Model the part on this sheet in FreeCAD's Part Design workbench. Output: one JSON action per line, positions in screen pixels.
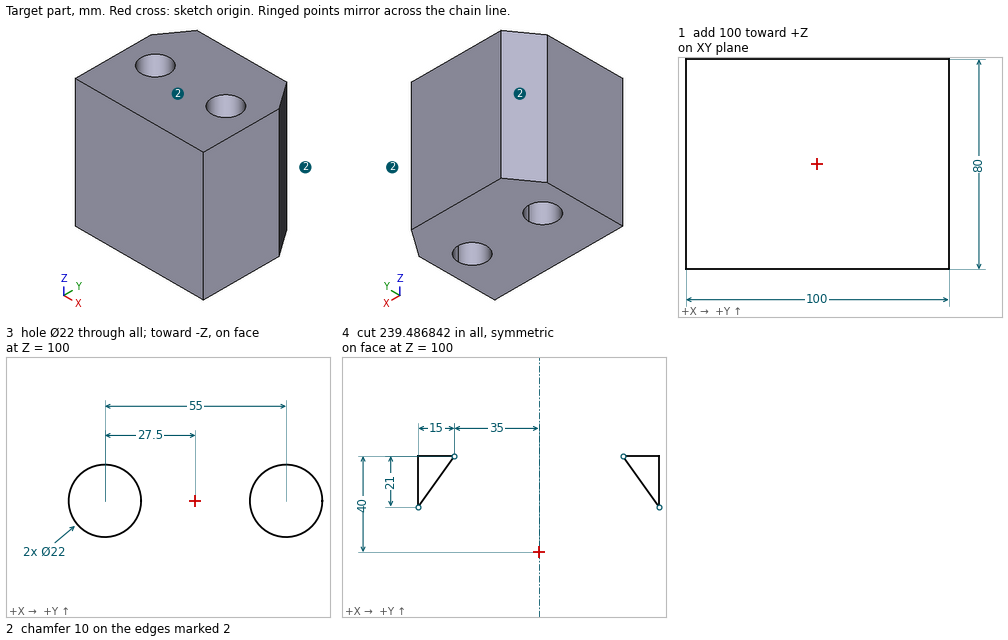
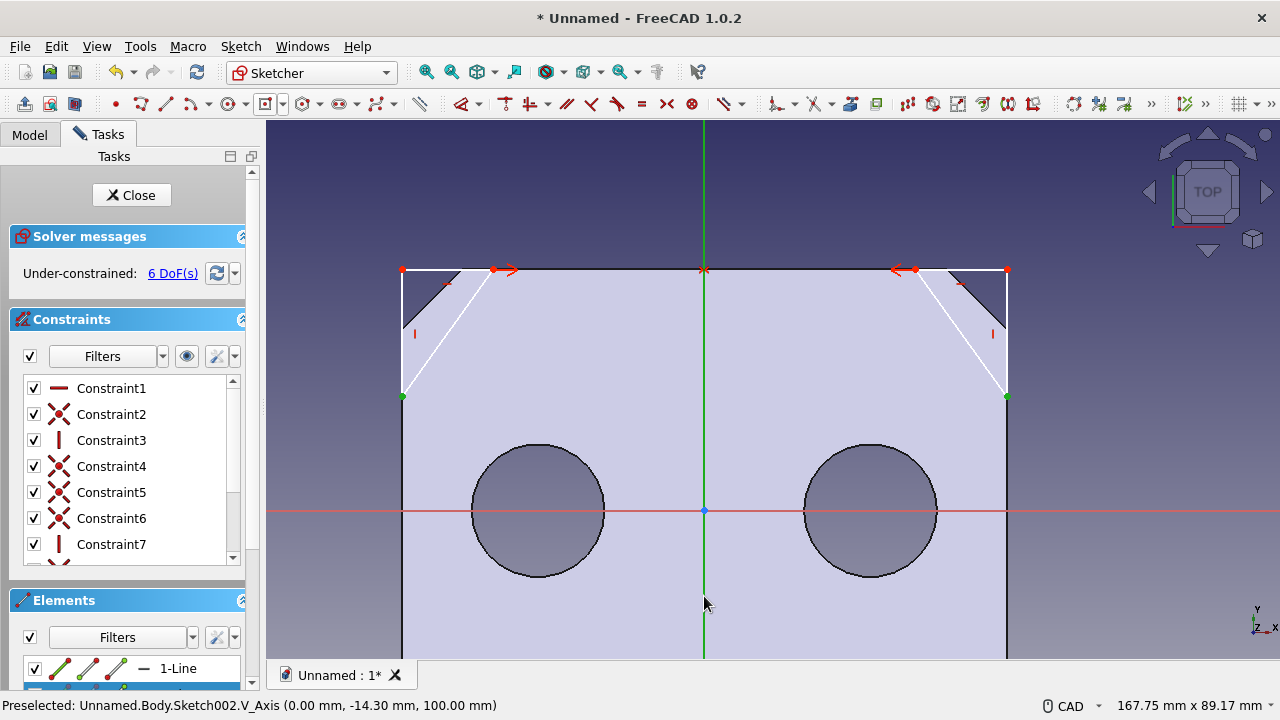
{"action": "left_click", "coordinate": [667, 104]}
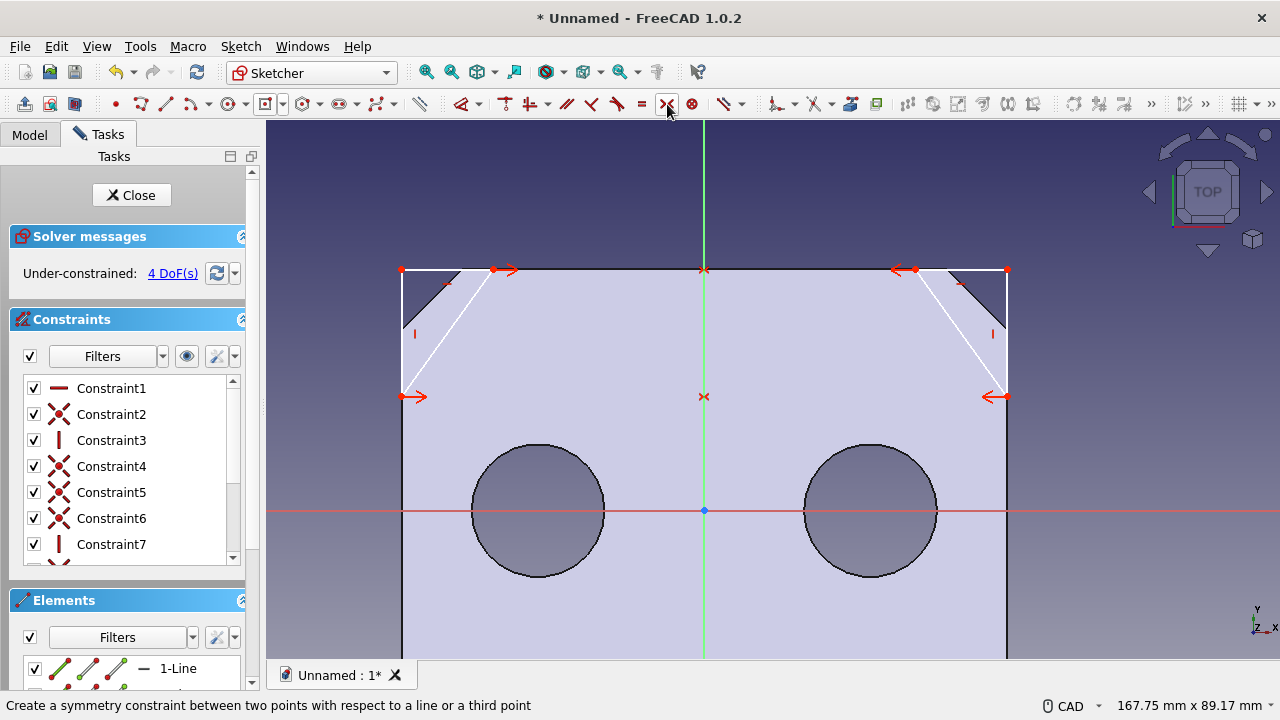
{"action": "left_click", "coordinate": [460, 104]}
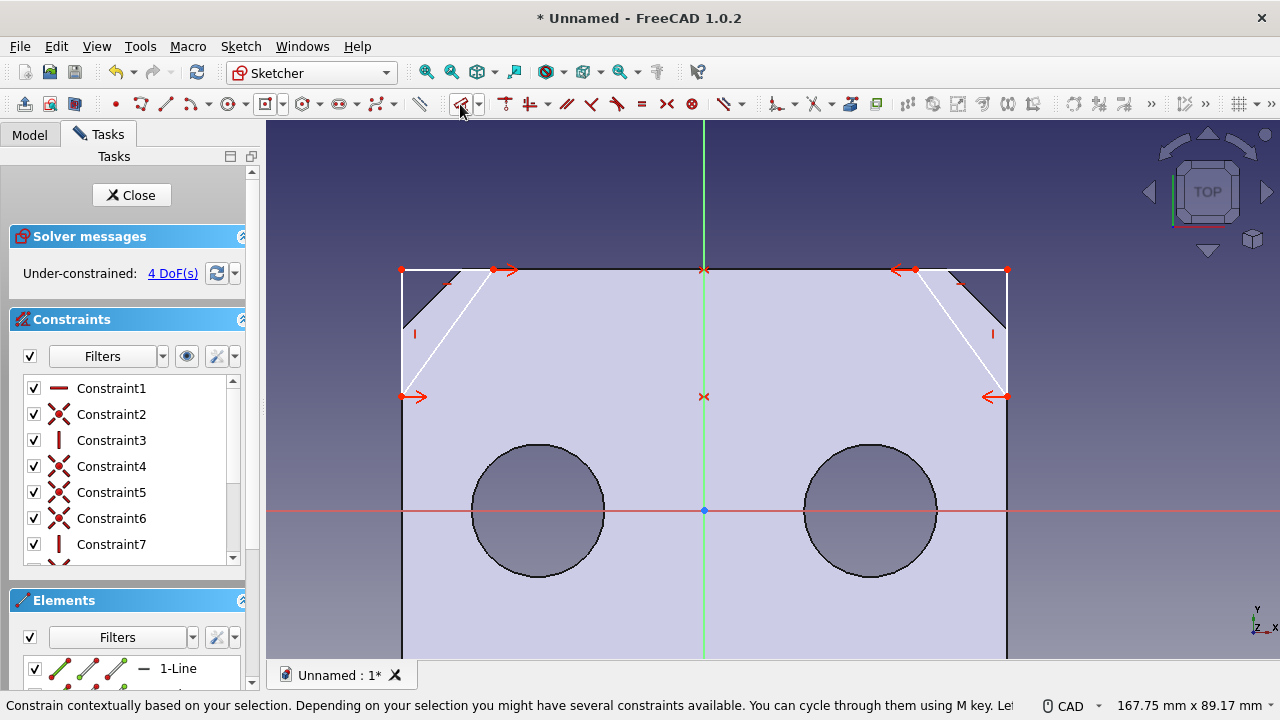
{"action": "left_click", "coordinate": [466, 270]}
{"action": "left_click", "coordinate": [447, 236]}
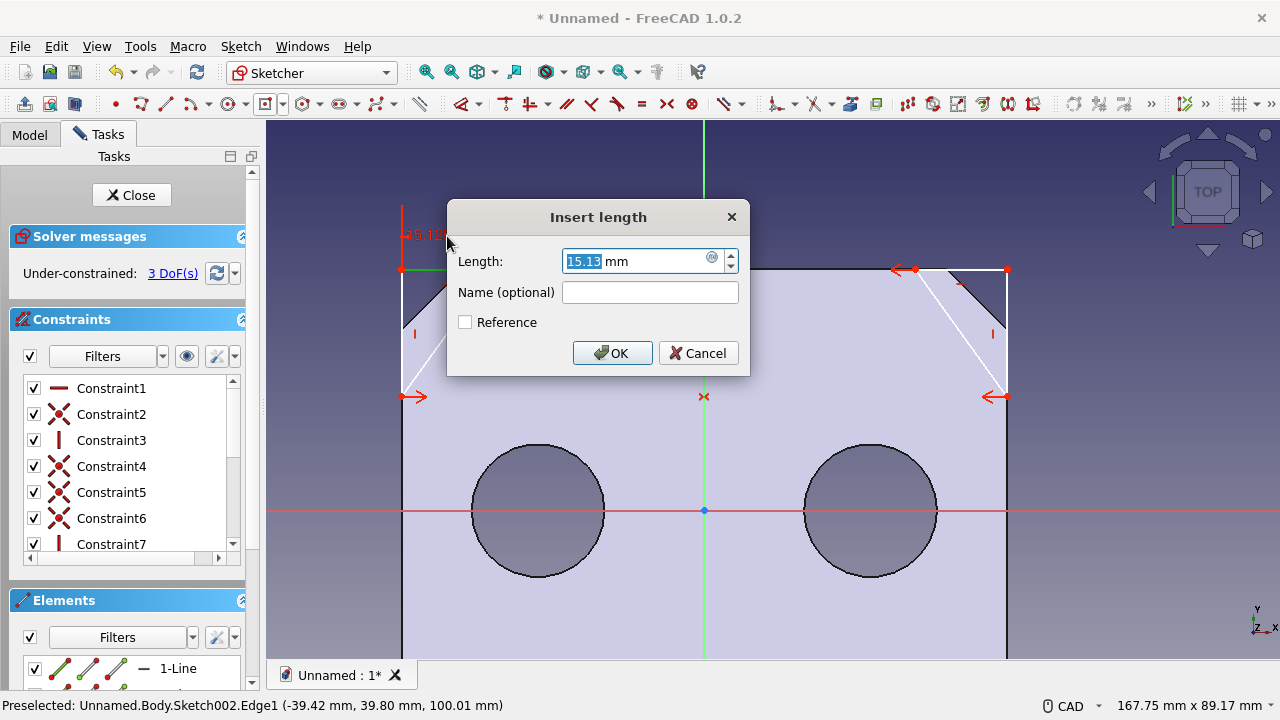
{"action": "type", "text": "15"}
{"action": "key", "text": "Return"}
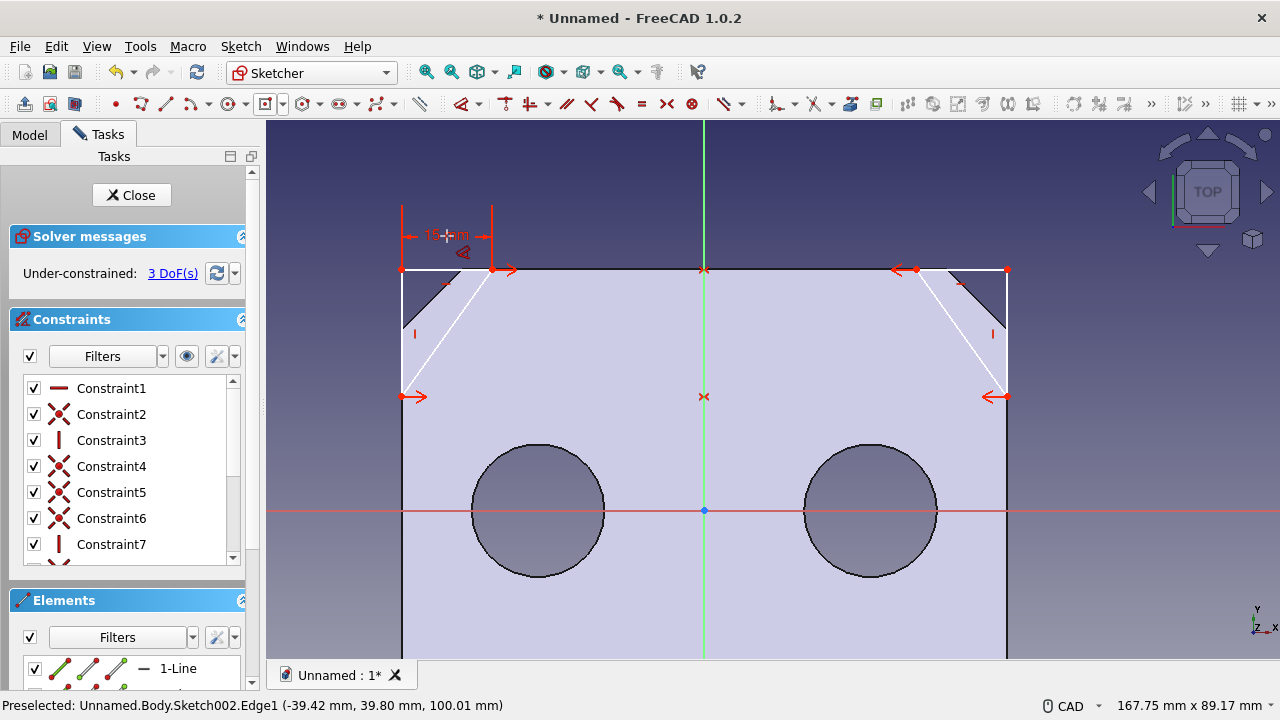
{"action": "left_click", "coordinate": [402, 308]}
{"action": "left_click", "coordinate": [368, 333]}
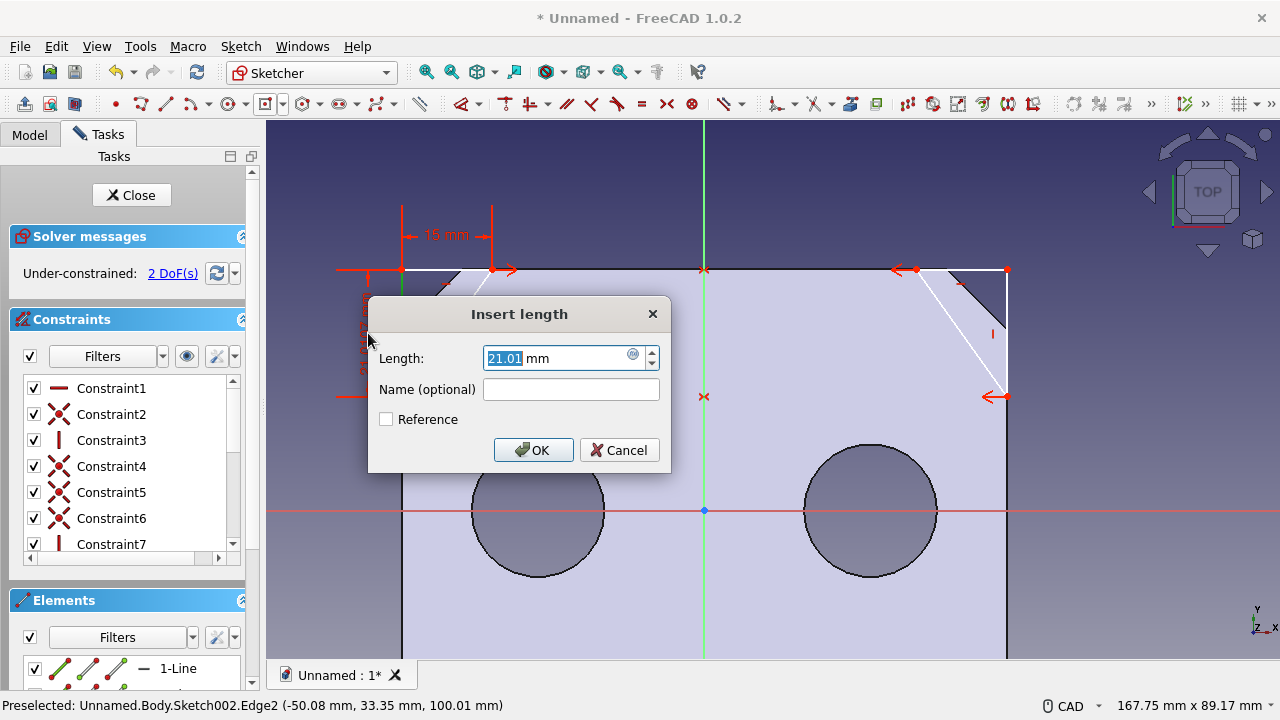
{"action": "type", "text": "21"}
{"action": "key", "text": "Return"}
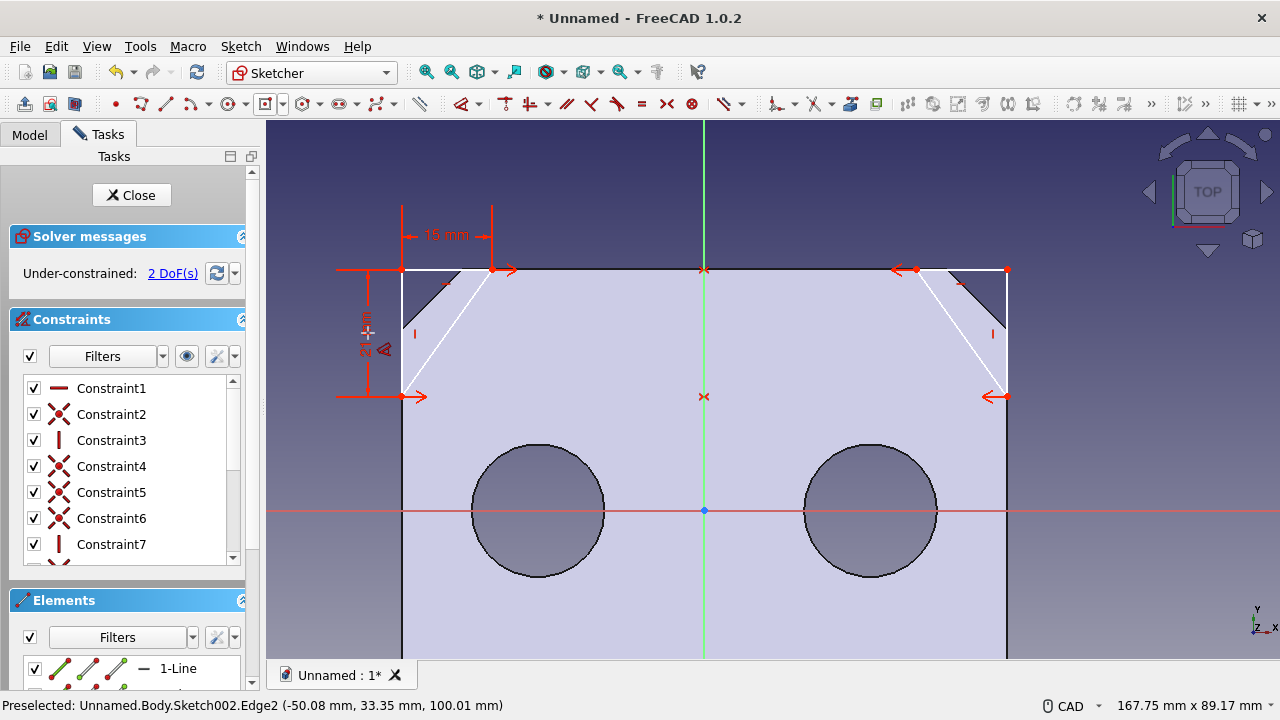
{"action": "left_click", "coordinate": [492, 270]}
{"action": "left_click", "coordinate": [598, 545]}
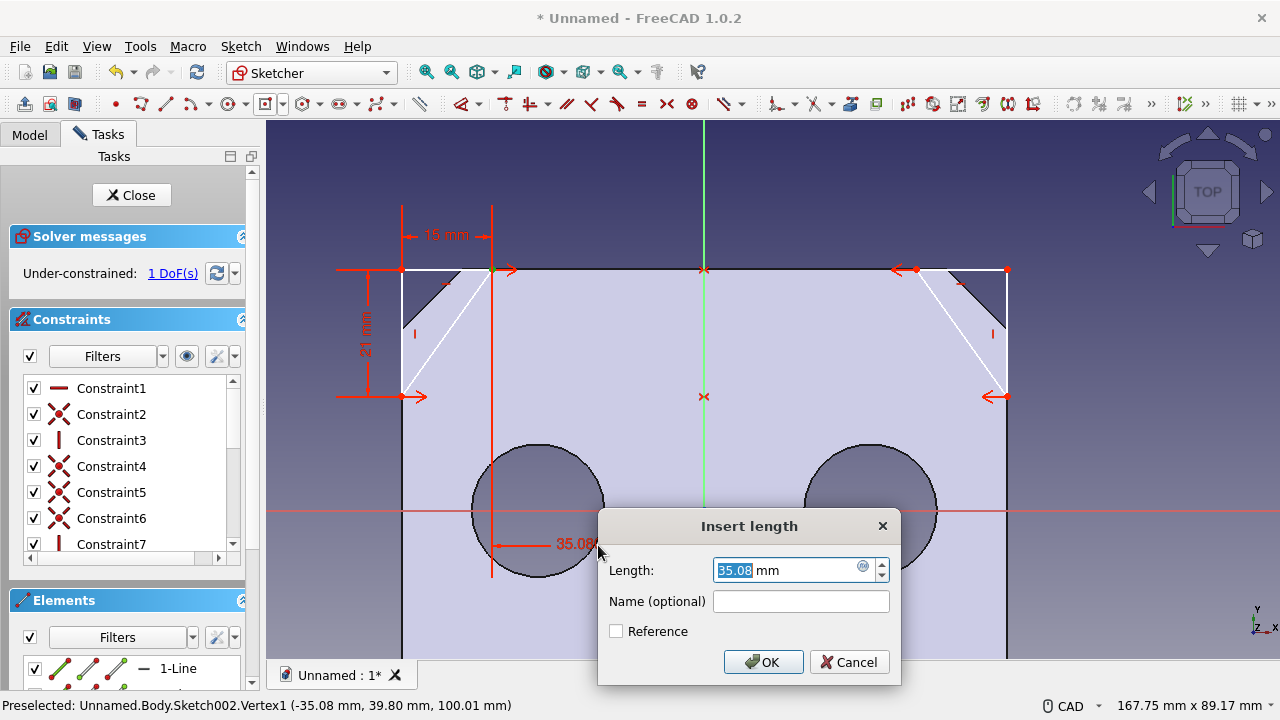
{"action": "type", "text": "35"}
{"action": "key", "text": "Return"}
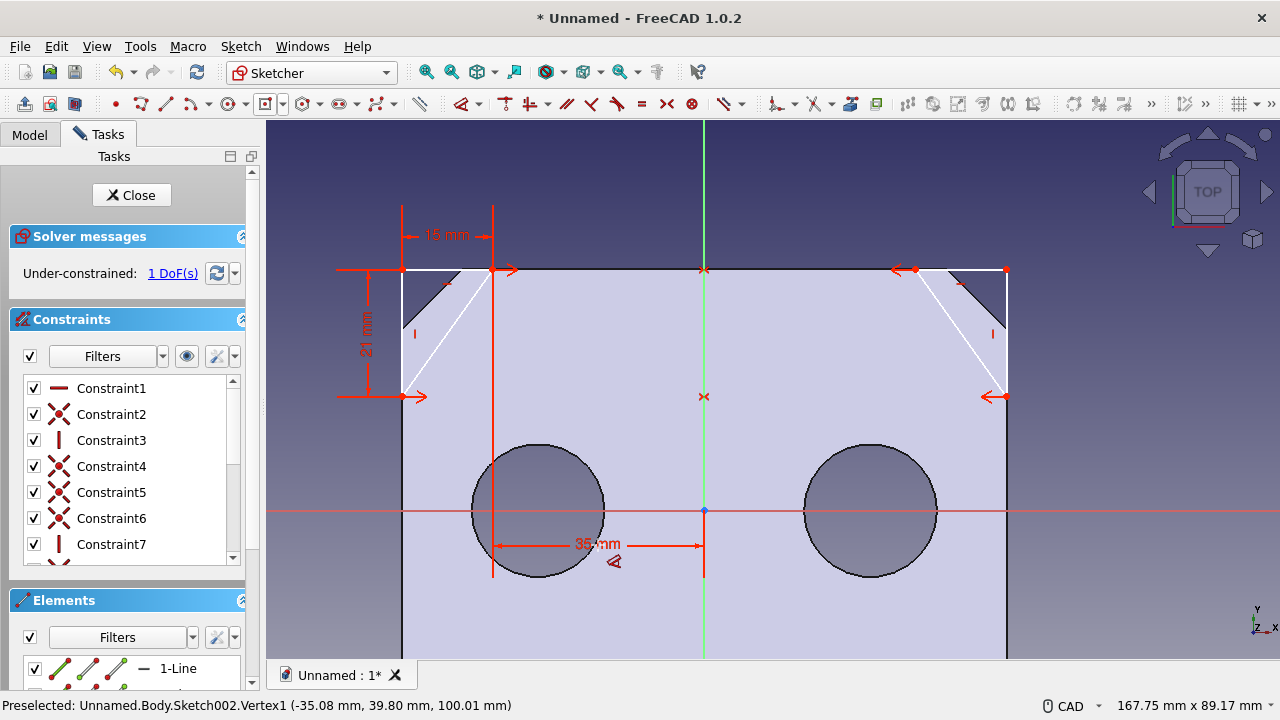
{"action": "left_click", "coordinate": [493, 270]}
{"action": "left_click", "coordinate": [459, 390]}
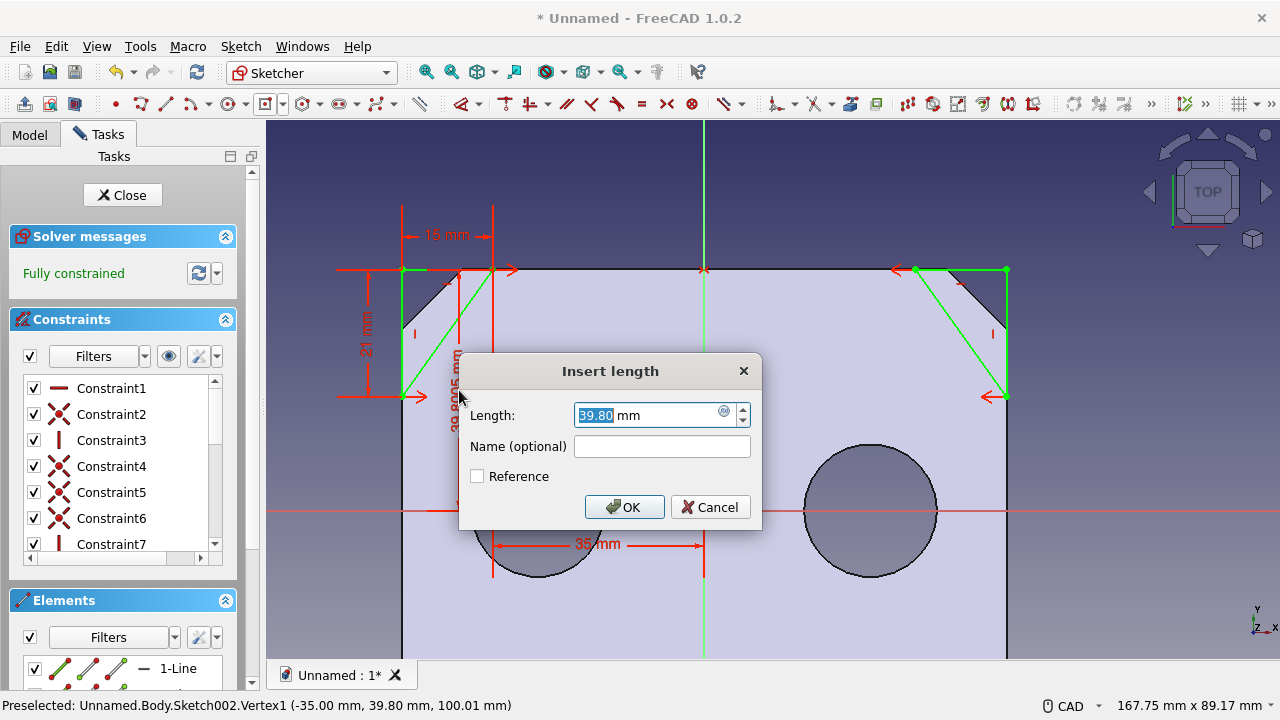
{"action": "type", "text": "40"}
{"action": "key", "text": "Return"}
{"action": "key", "text": "Escape"}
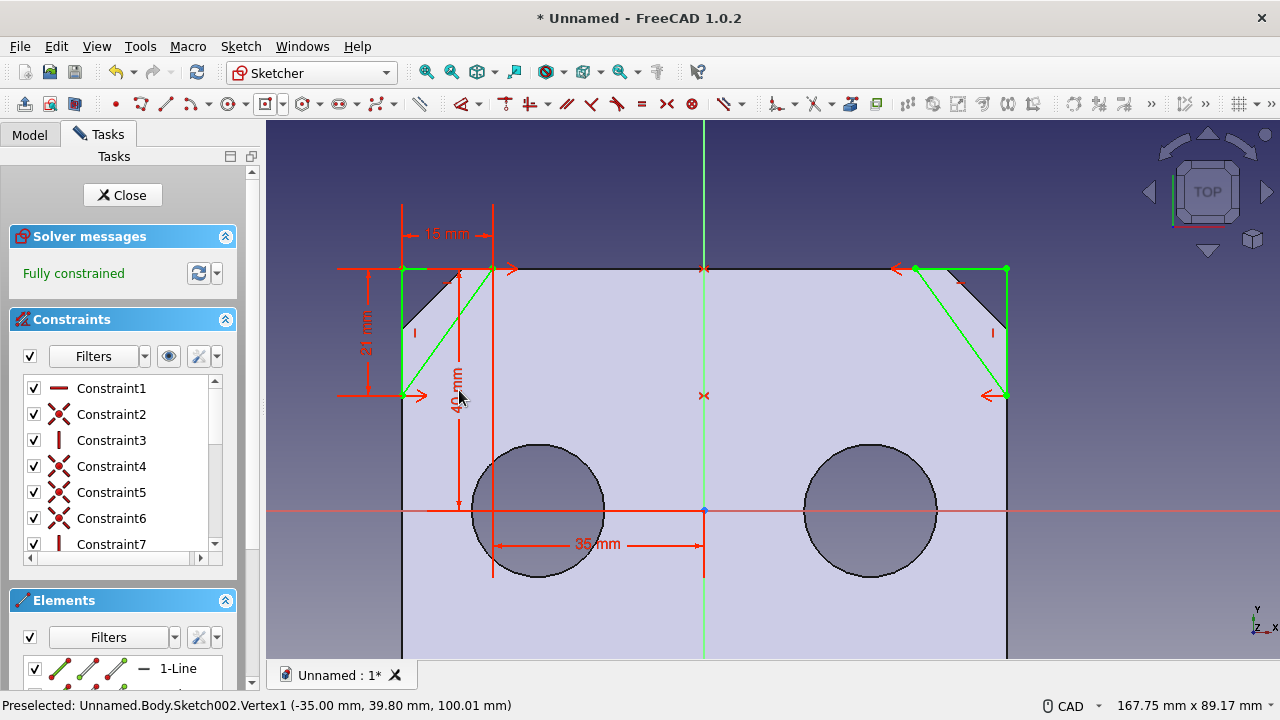
{"action": "left_click", "coordinate": [123, 195]}